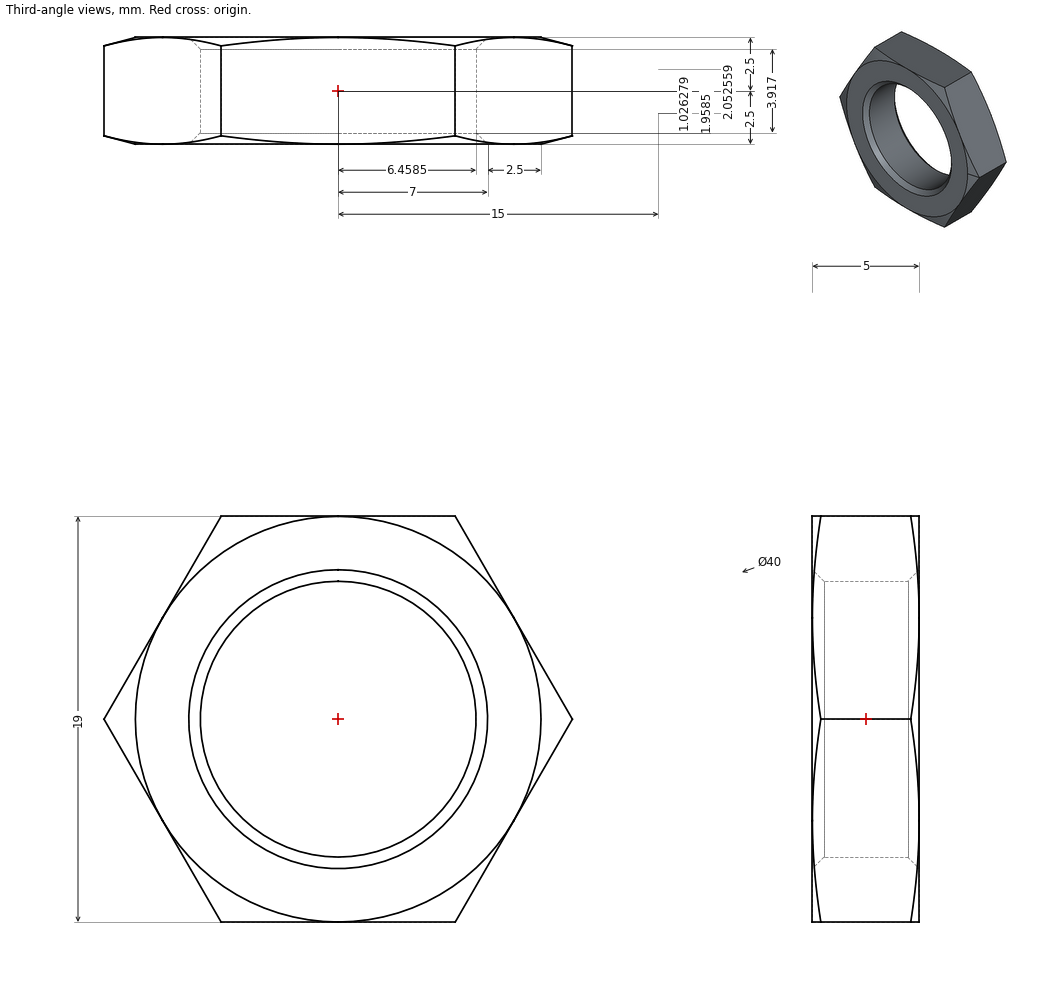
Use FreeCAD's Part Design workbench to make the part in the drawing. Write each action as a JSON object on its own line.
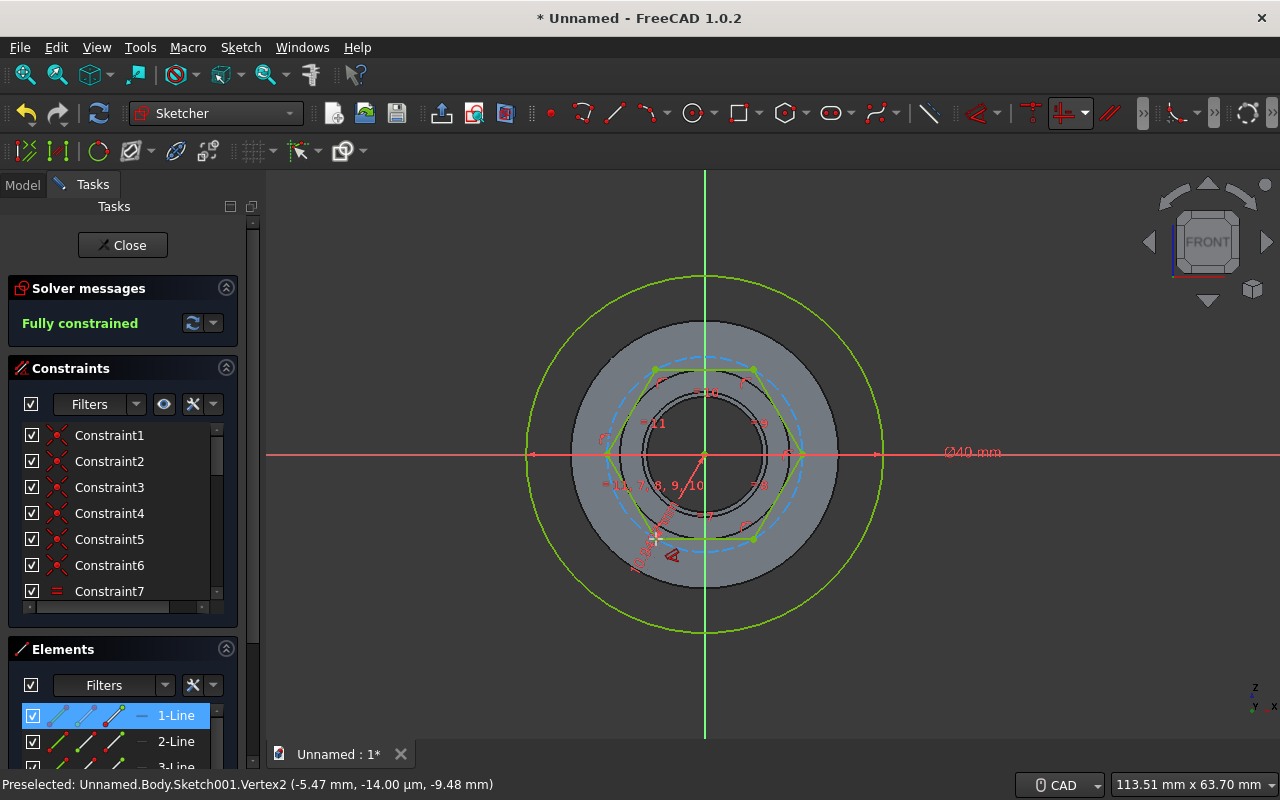
{"action": "left_click", "coordinate": [754, 370]}
{"action": "left_click", "coordinate": [812, 416]}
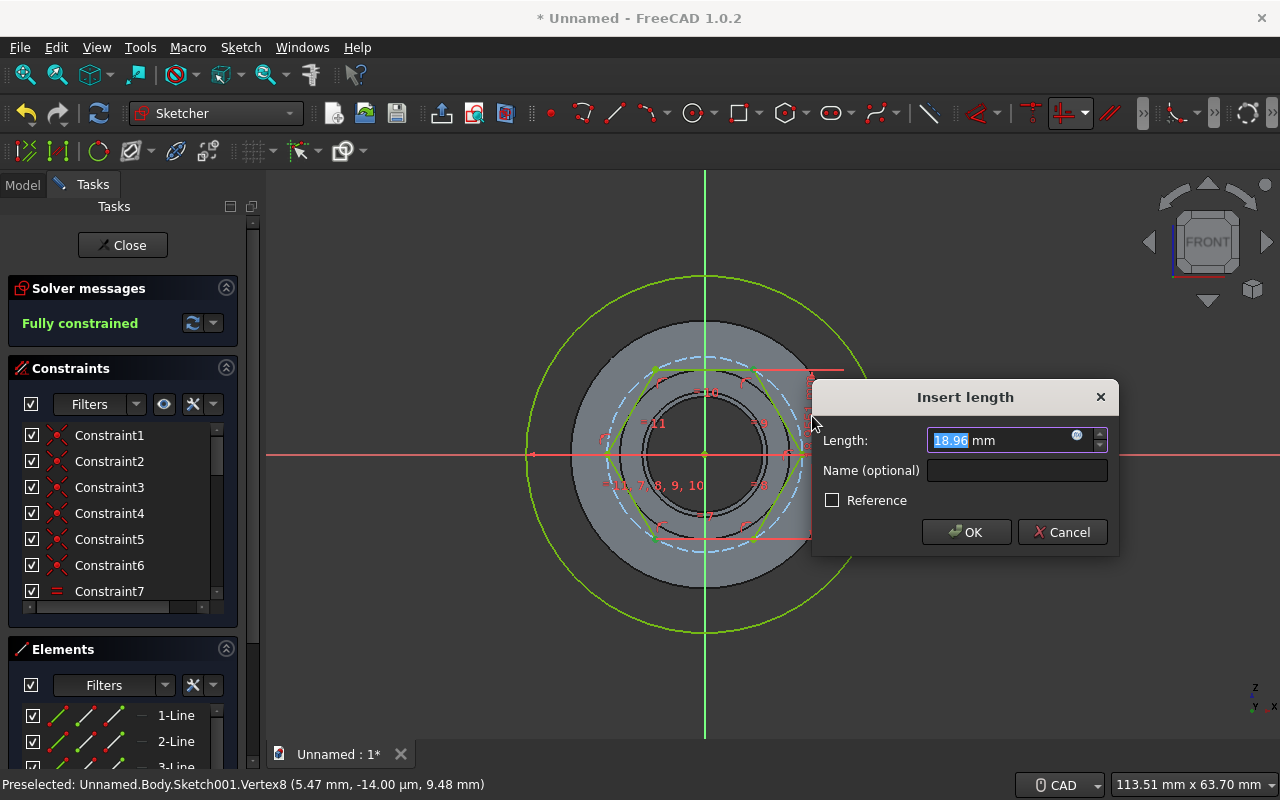
{"action": "type", "text": "19"}
{"action": "key", "text": "Return"}
{"action": "key", "text": "Escape"}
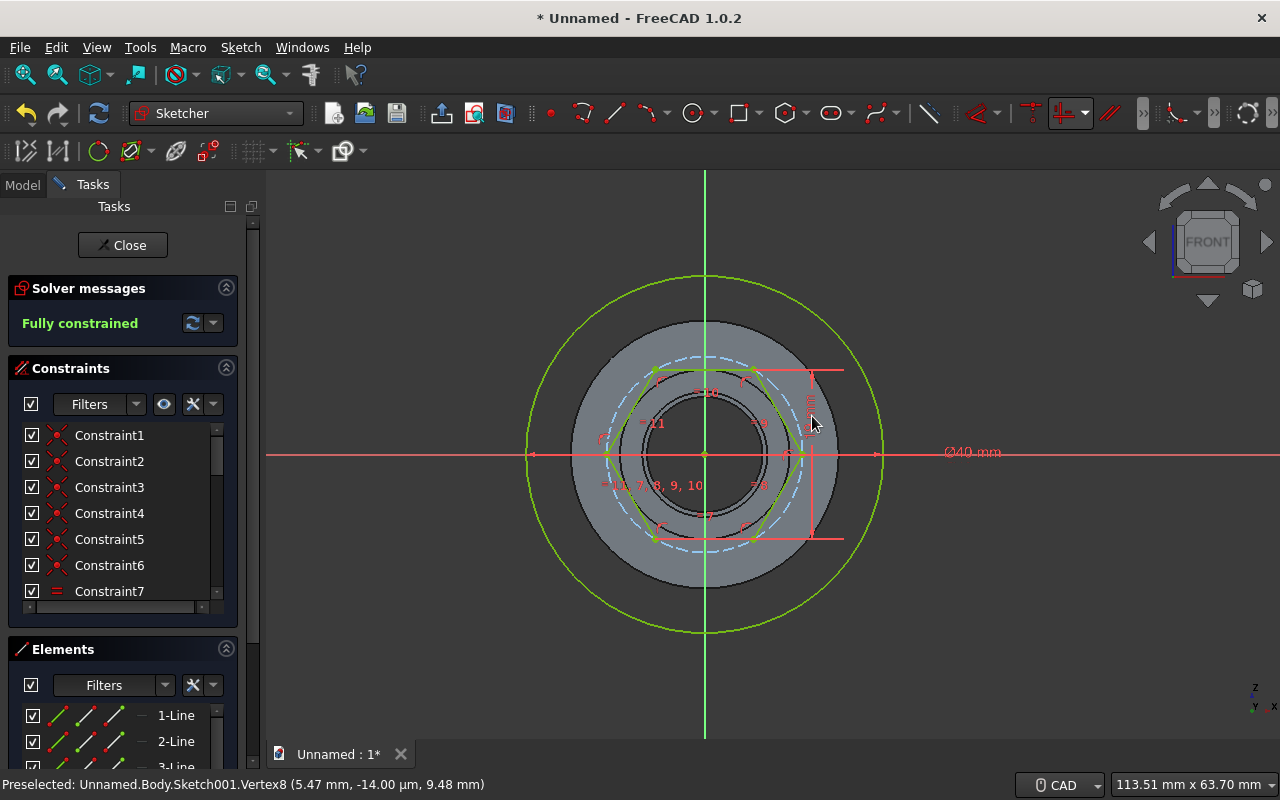
{"action": "left_click", "coordinate": [123, 245]}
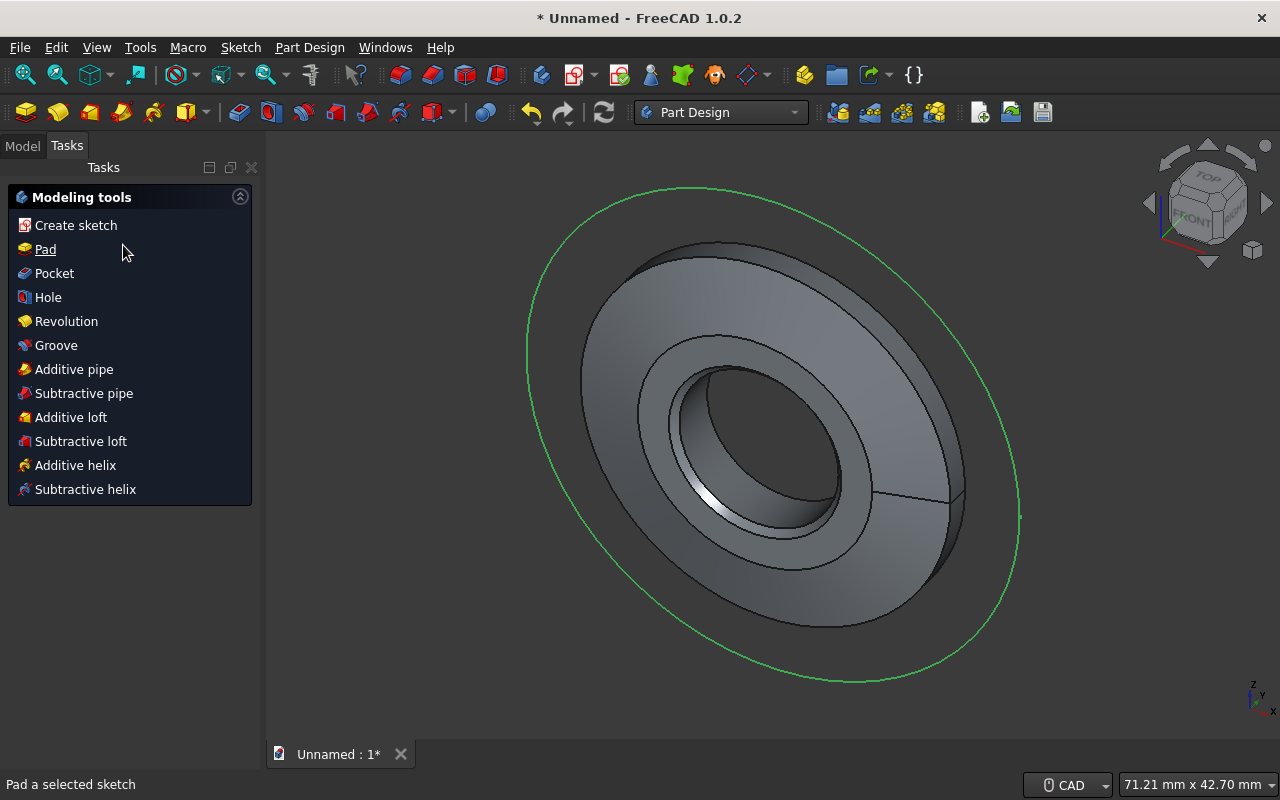
{"action": "left_click", "coordinate": [240, 112]}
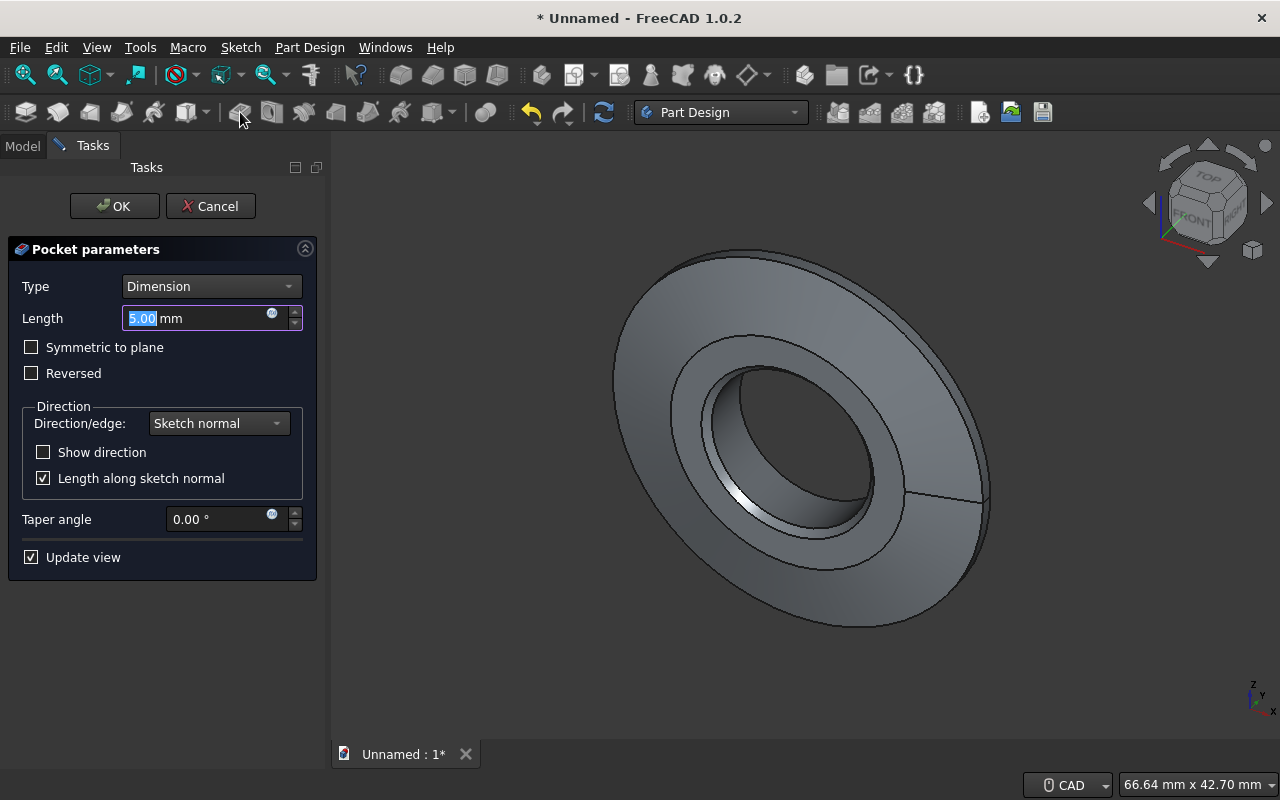
{"action": "type", "text": "5"}
{"action": "key", "text": "Tab"}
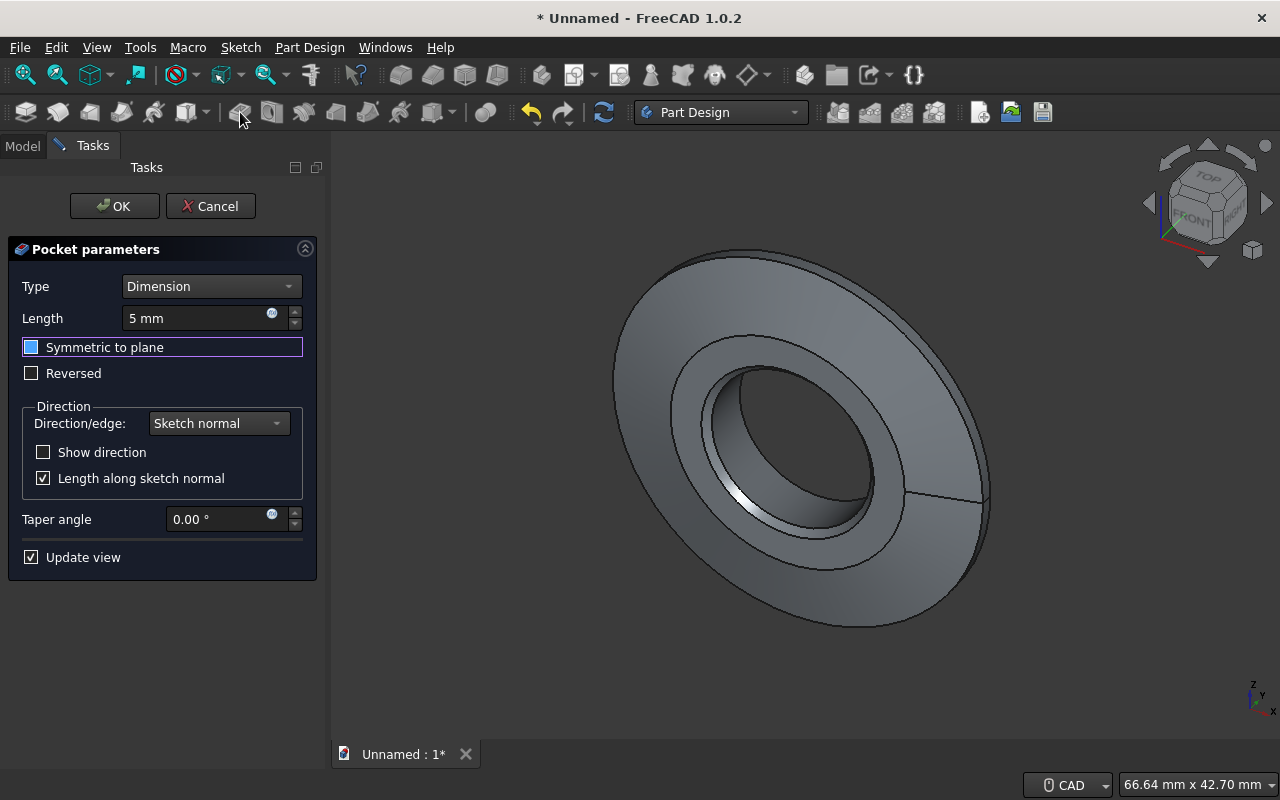
{"action": "left_click", "coordinate": [30, 347]}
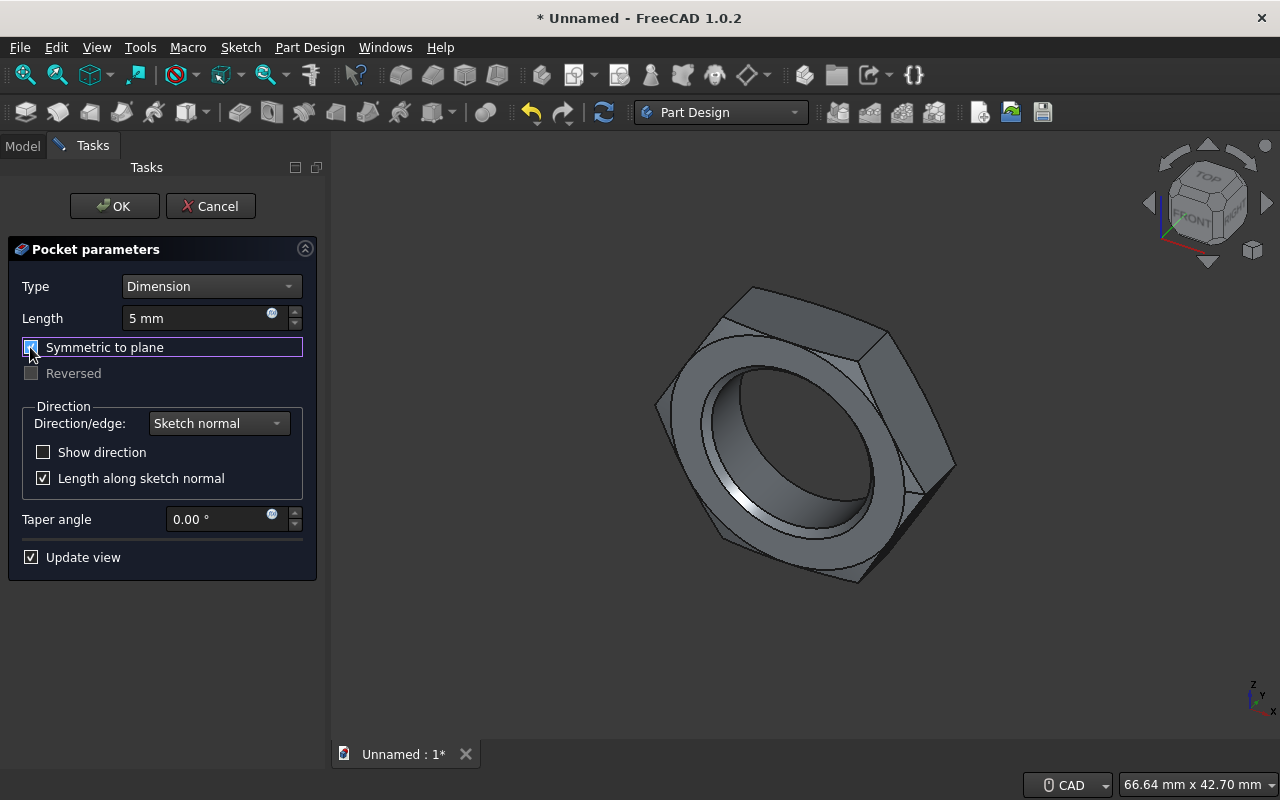
{"action": "left_click", "coordinate": [115, 206]}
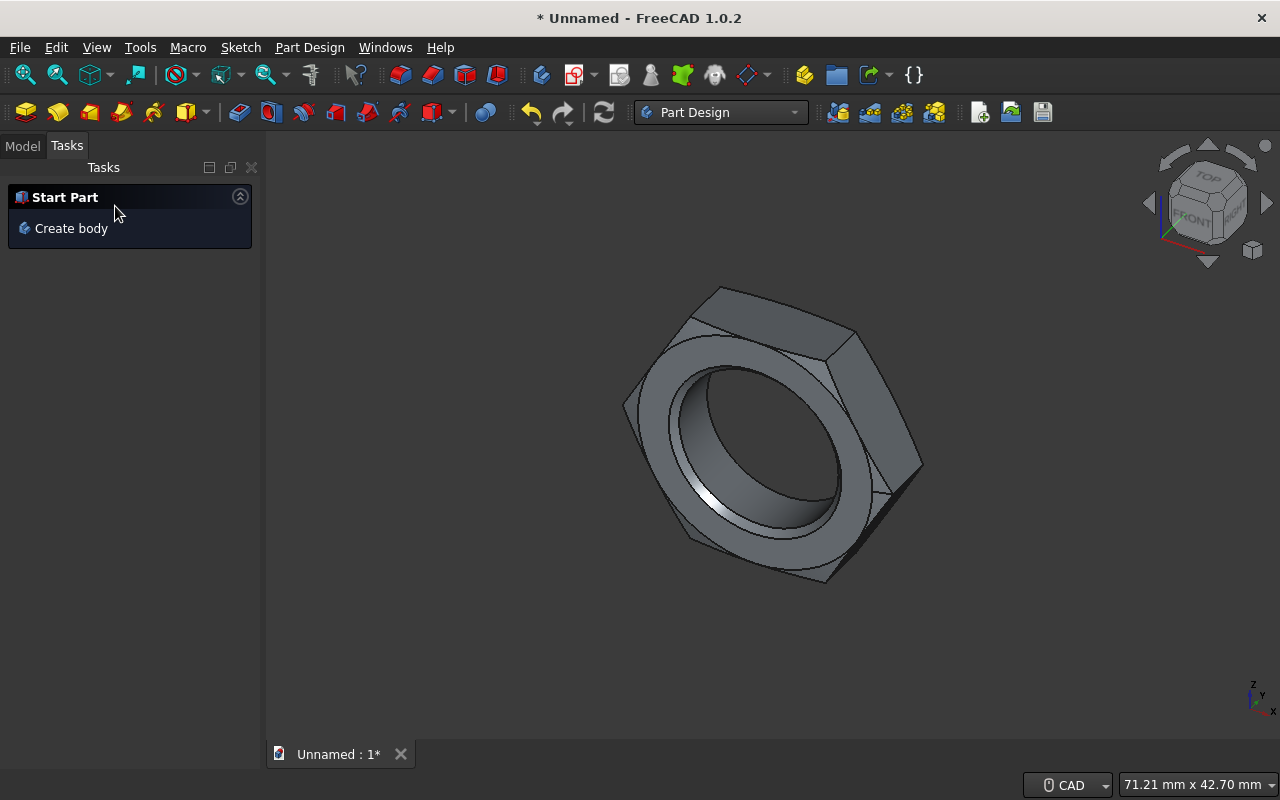
{"action": "key", "text": "0"}